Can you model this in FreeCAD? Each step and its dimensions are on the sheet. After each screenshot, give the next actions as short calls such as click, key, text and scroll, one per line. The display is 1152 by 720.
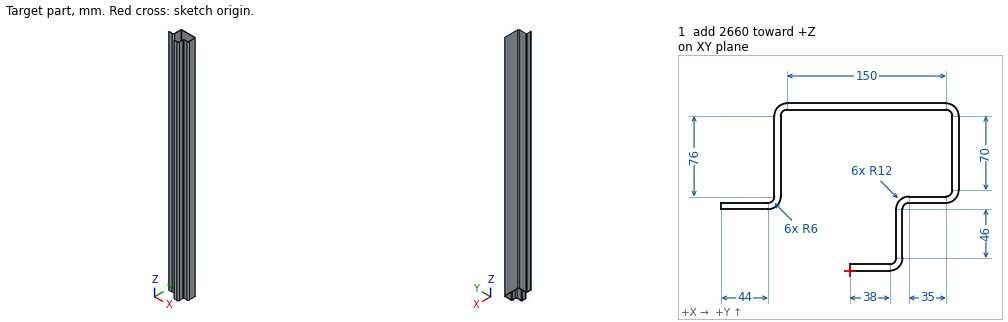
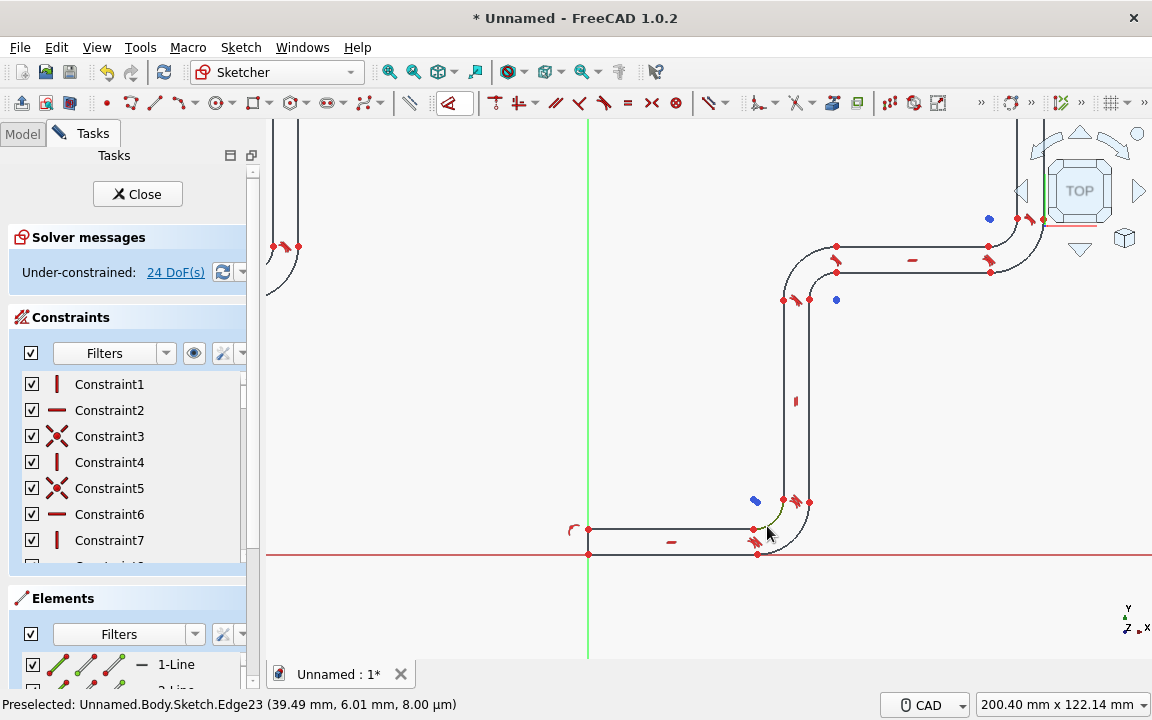
click(804, 526)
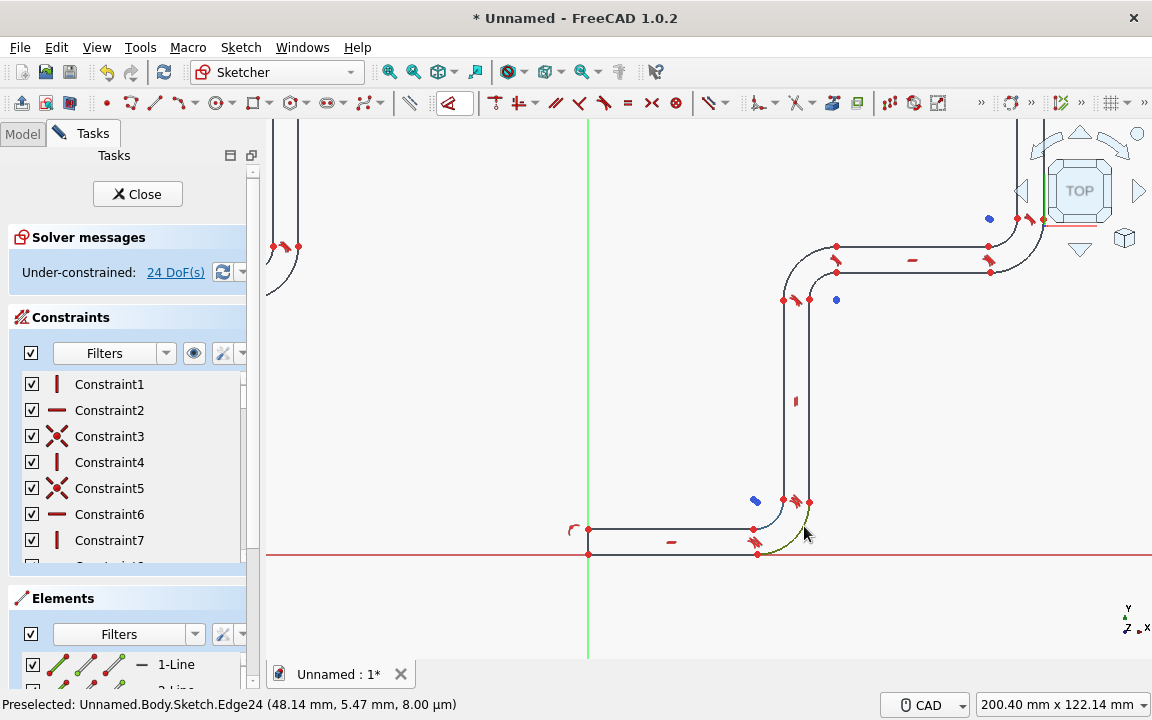
key(c)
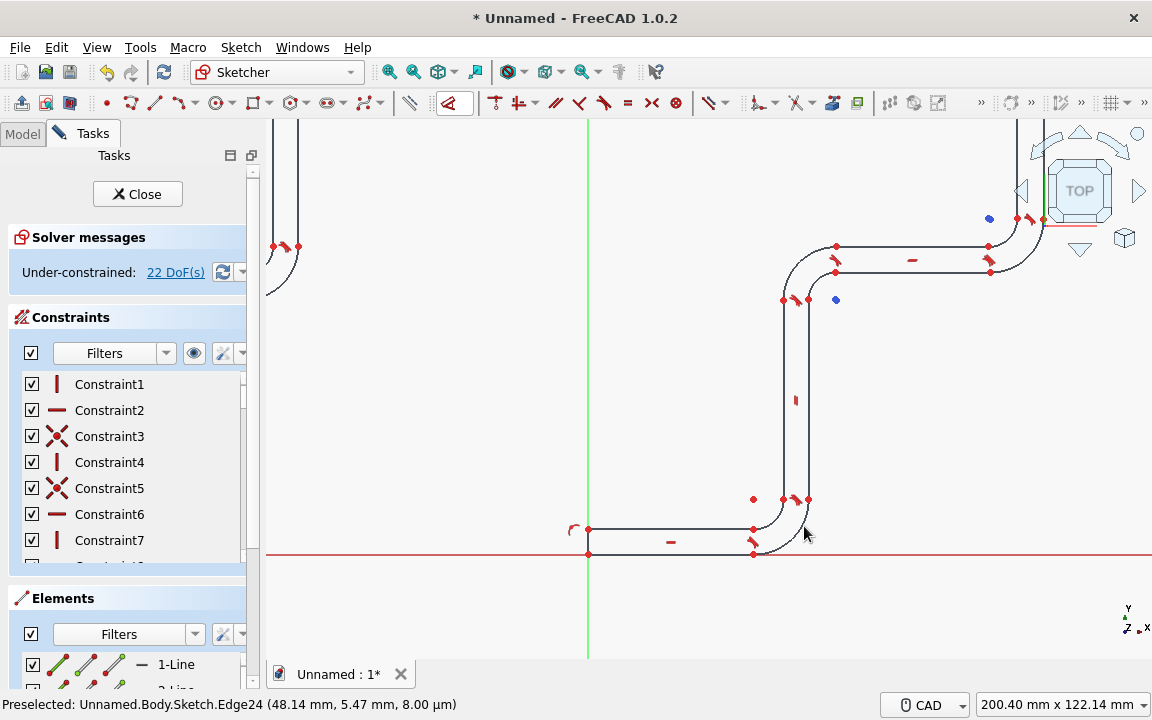
click(813, 253)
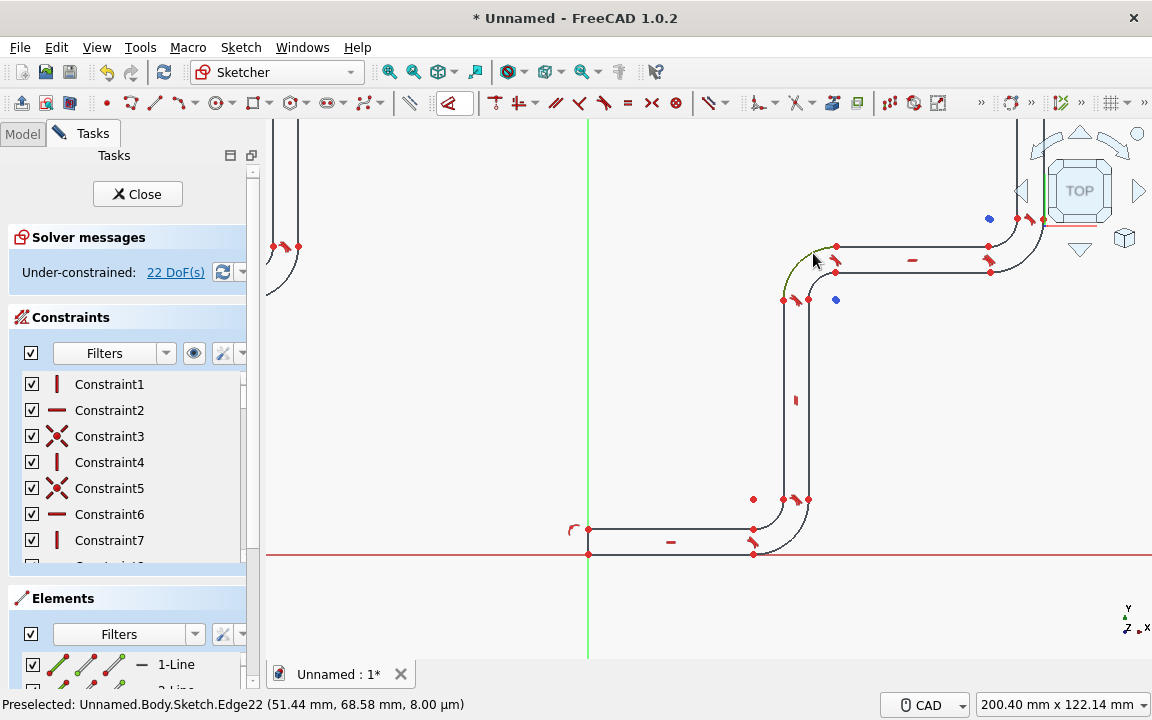
click(823, 276)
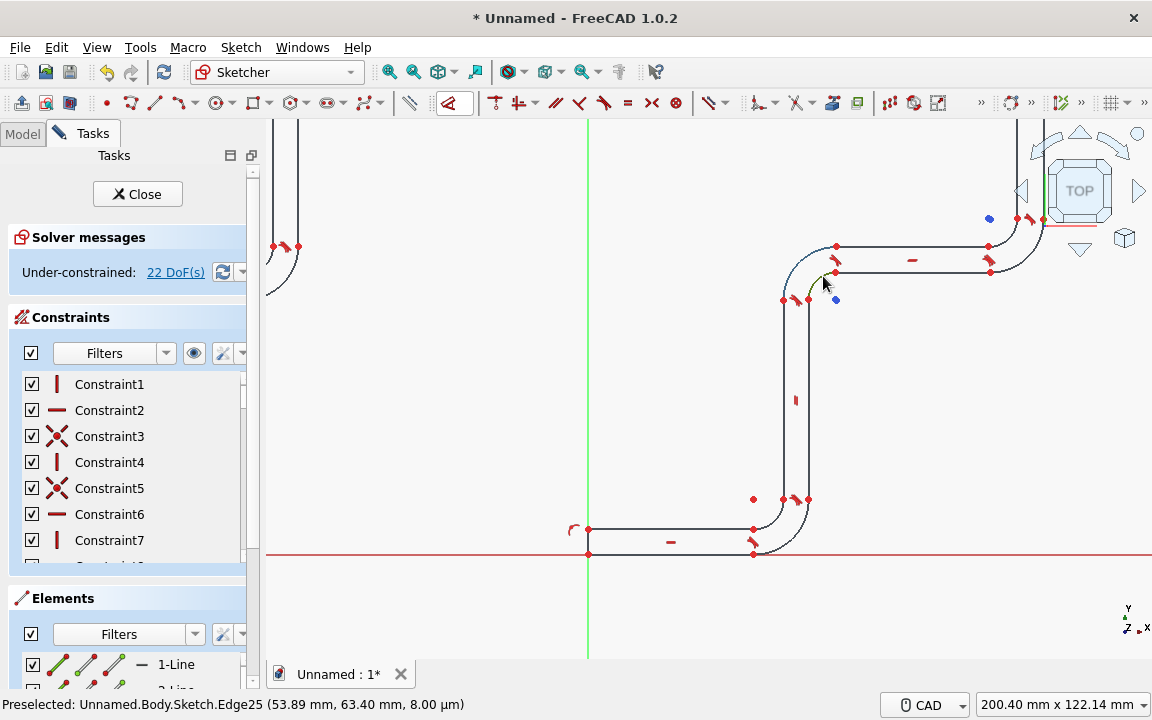
key(c)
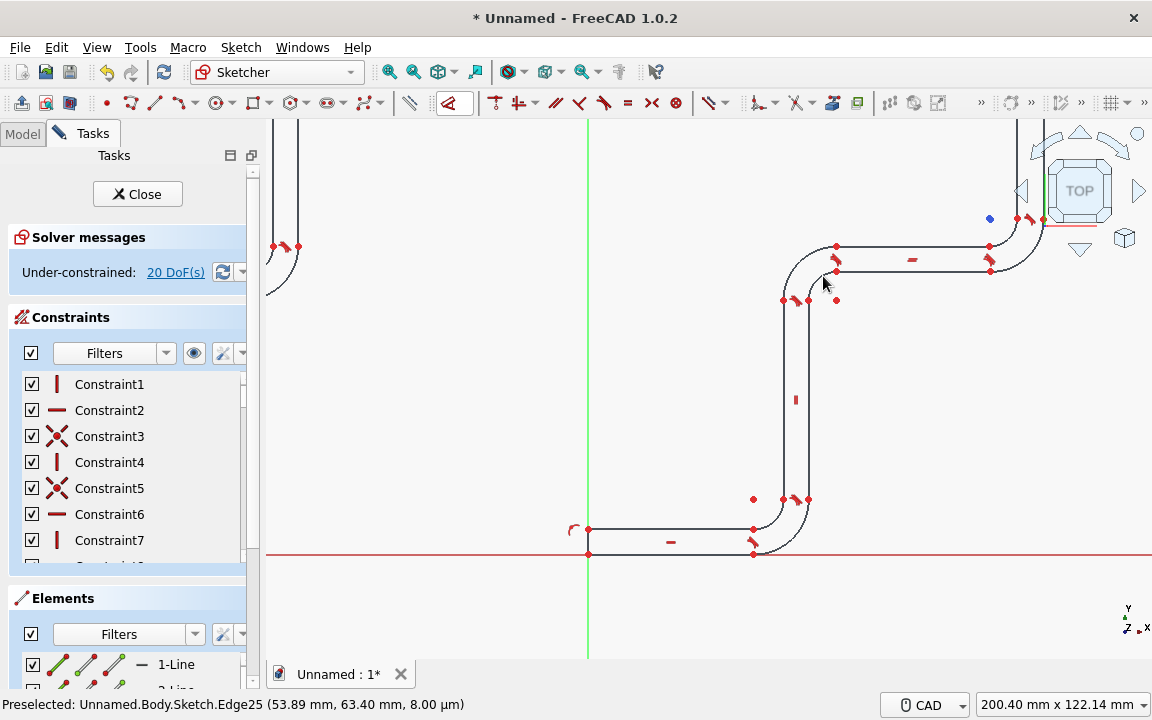
scroll(716, 539, down, 4)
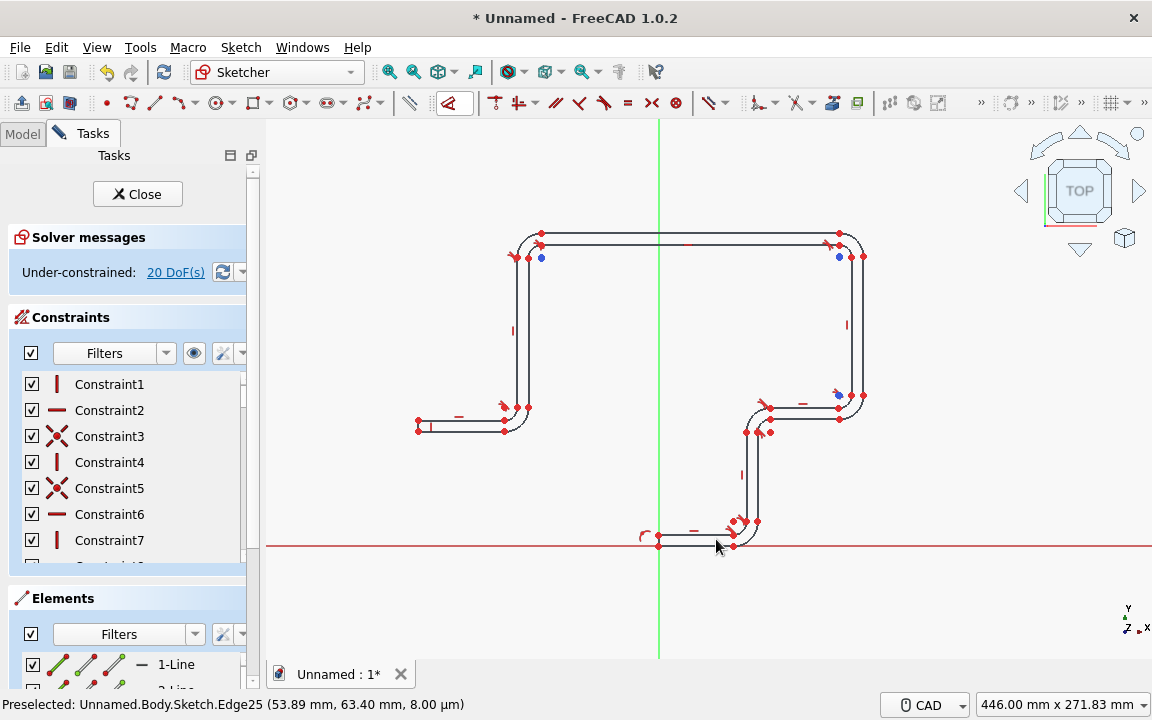
scroll(845, 407, up, 5)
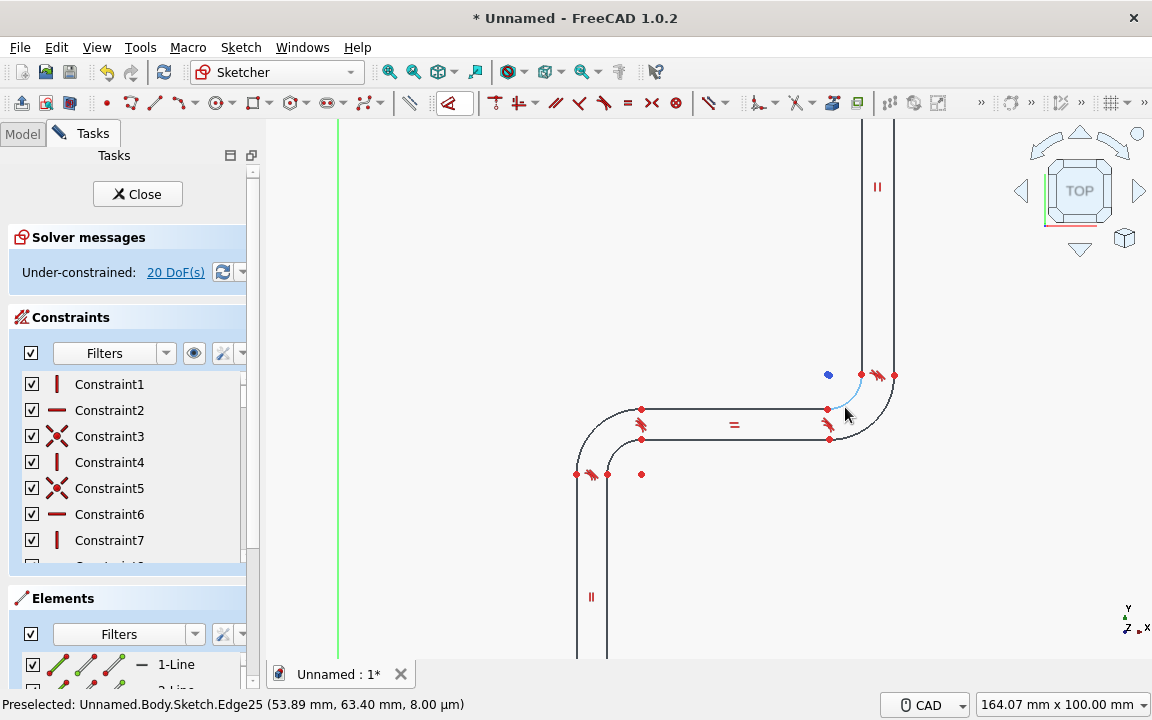
click(843, 405)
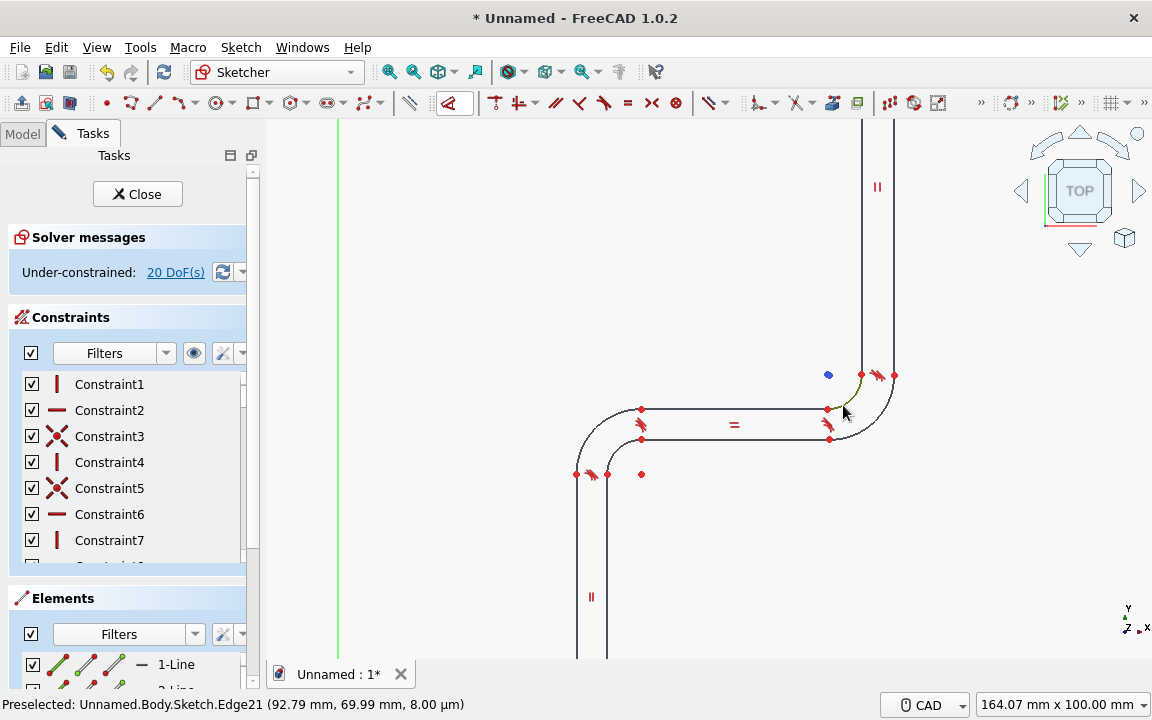
click(859, 433)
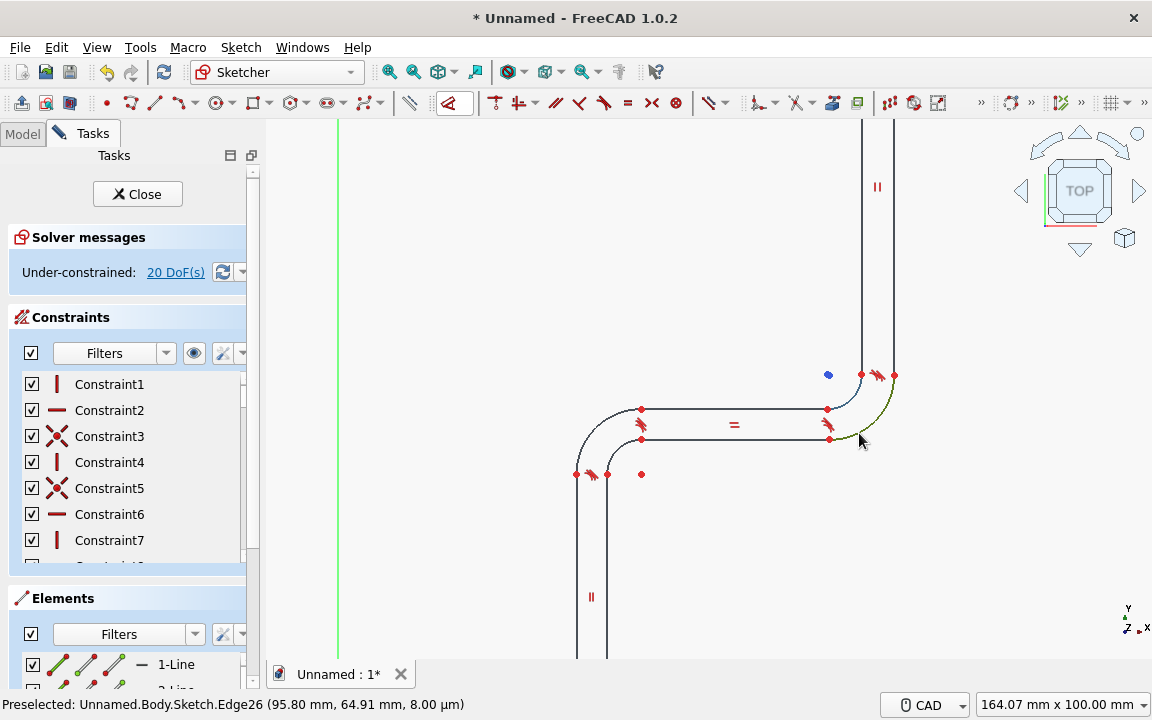
key(c)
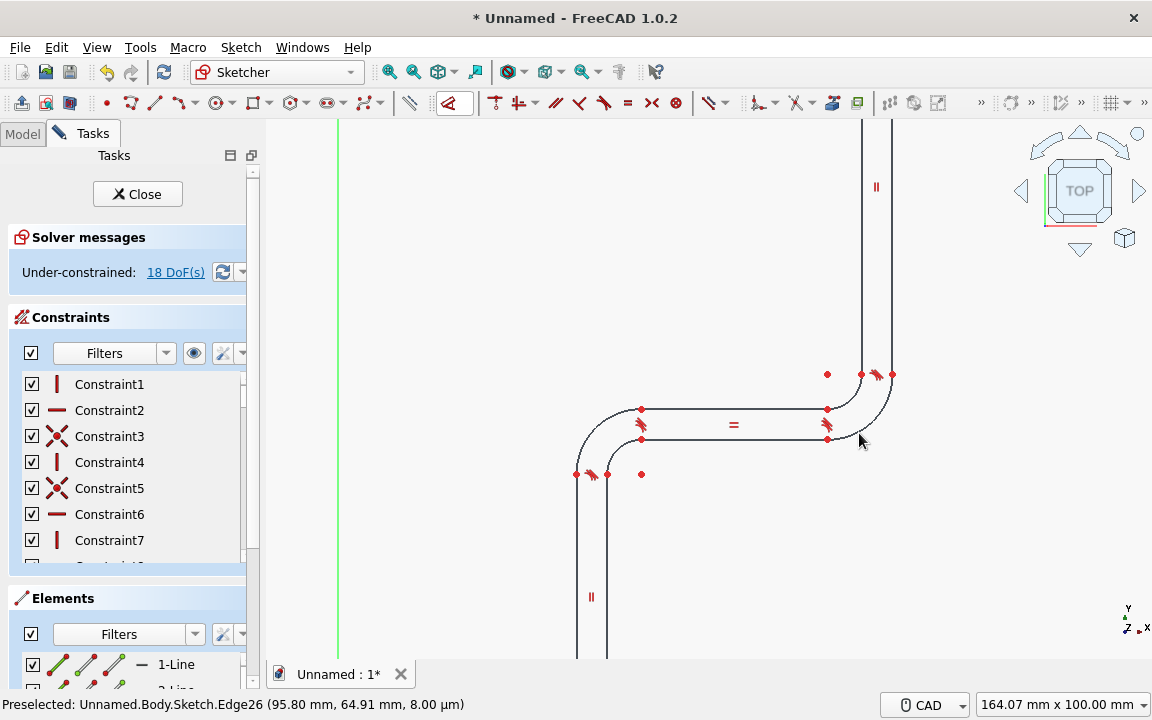
scroll(845, 407, down, 5)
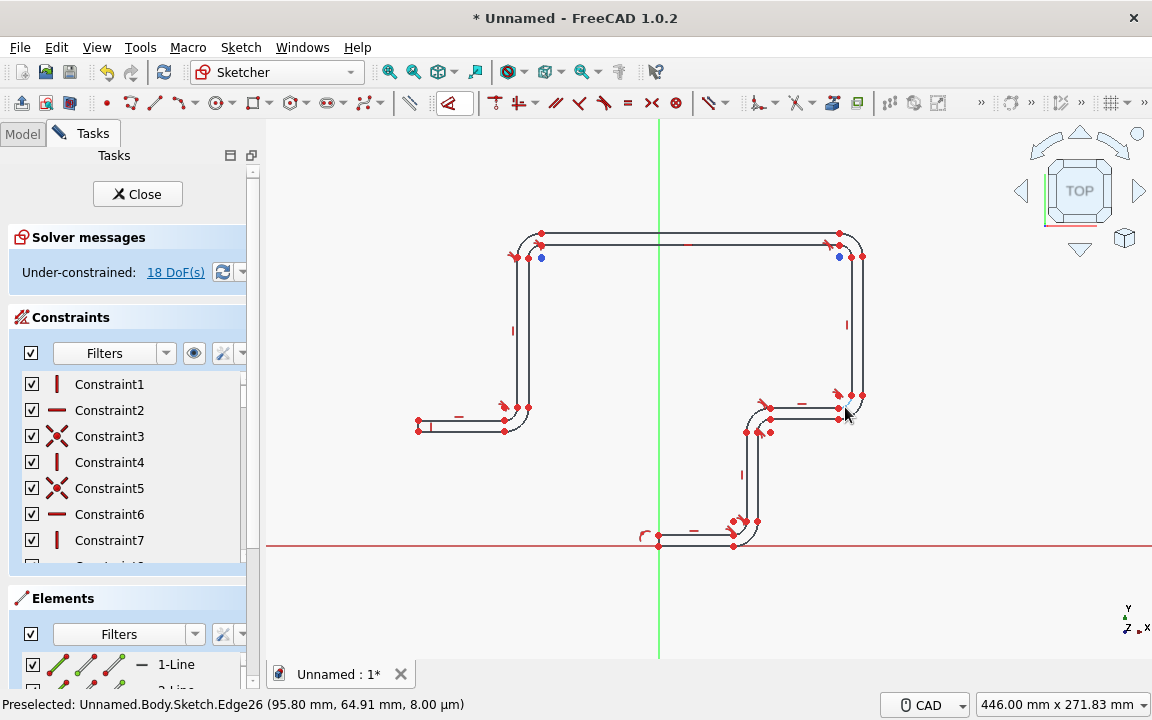
scroll(850, 252, up, 5)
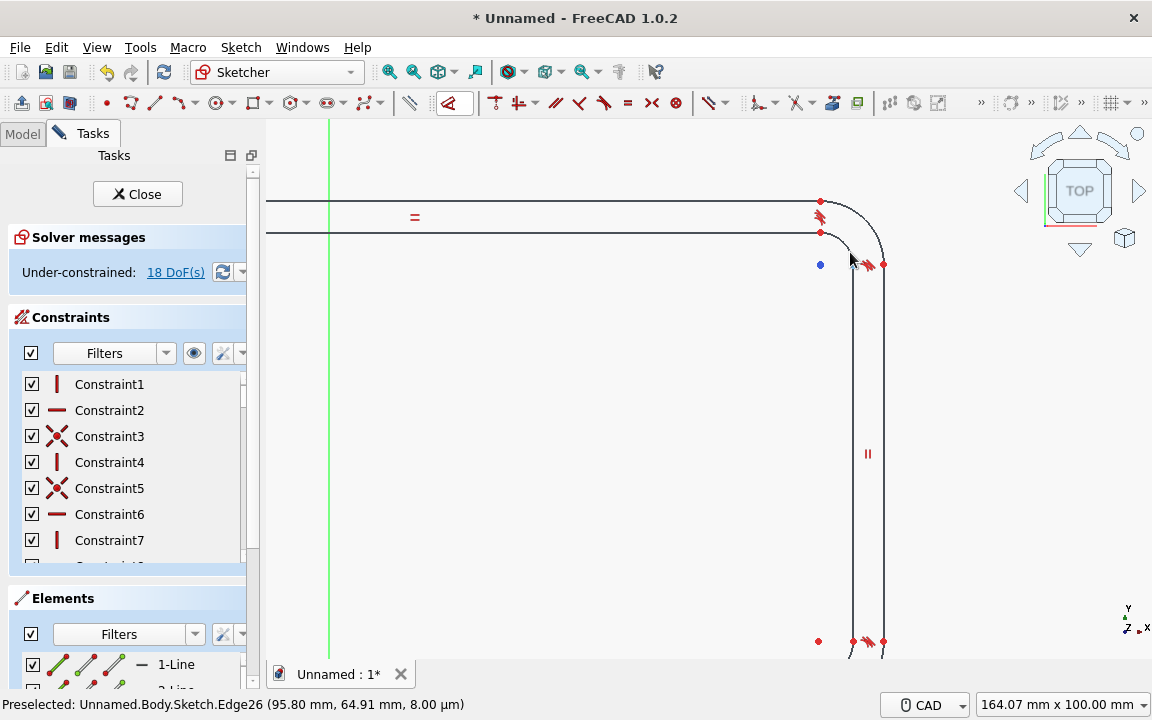
click(850, 251)